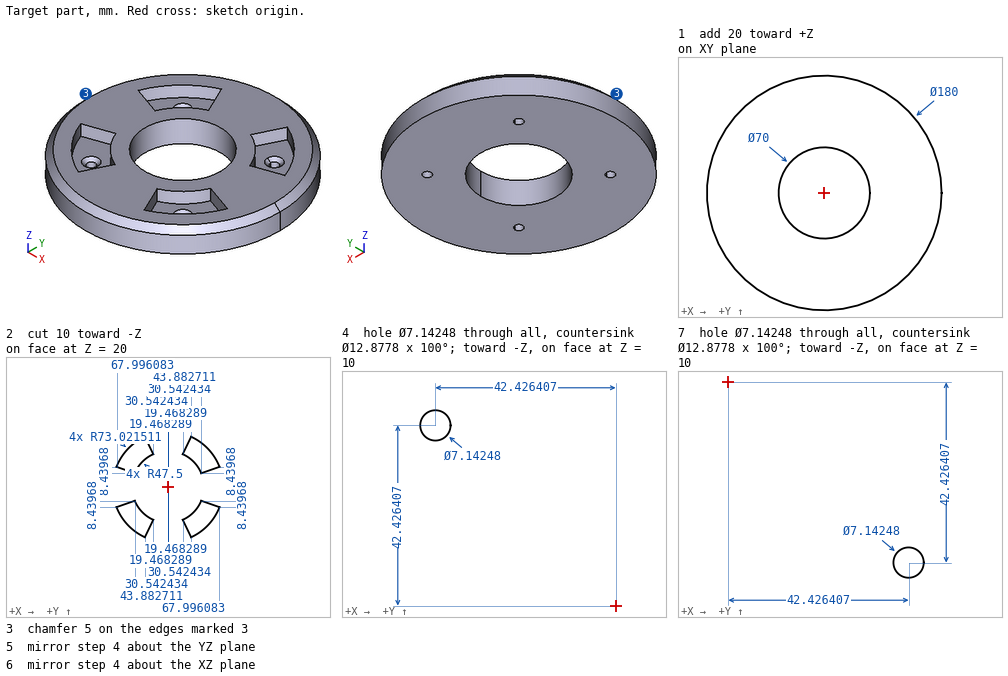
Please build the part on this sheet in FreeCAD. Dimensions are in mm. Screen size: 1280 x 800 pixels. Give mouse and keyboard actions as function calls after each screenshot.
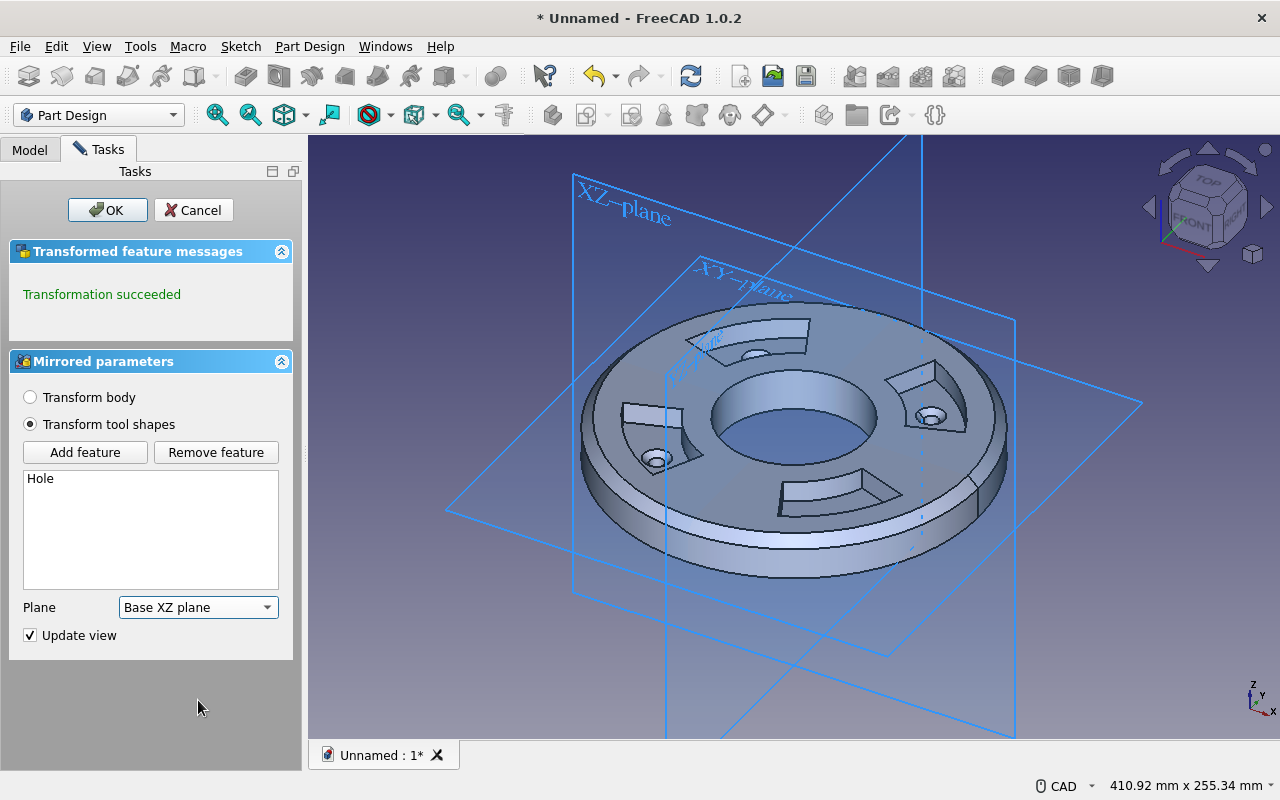
click(108, 210)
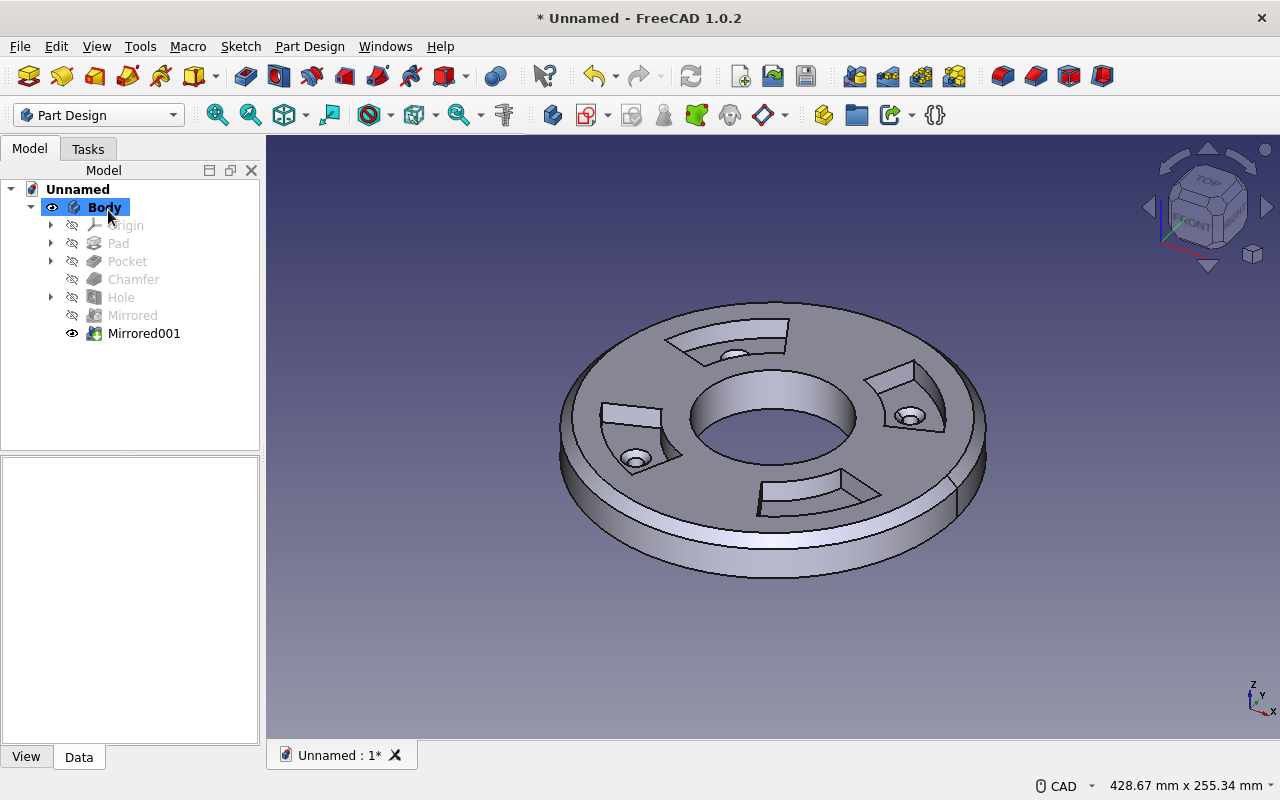
key(0)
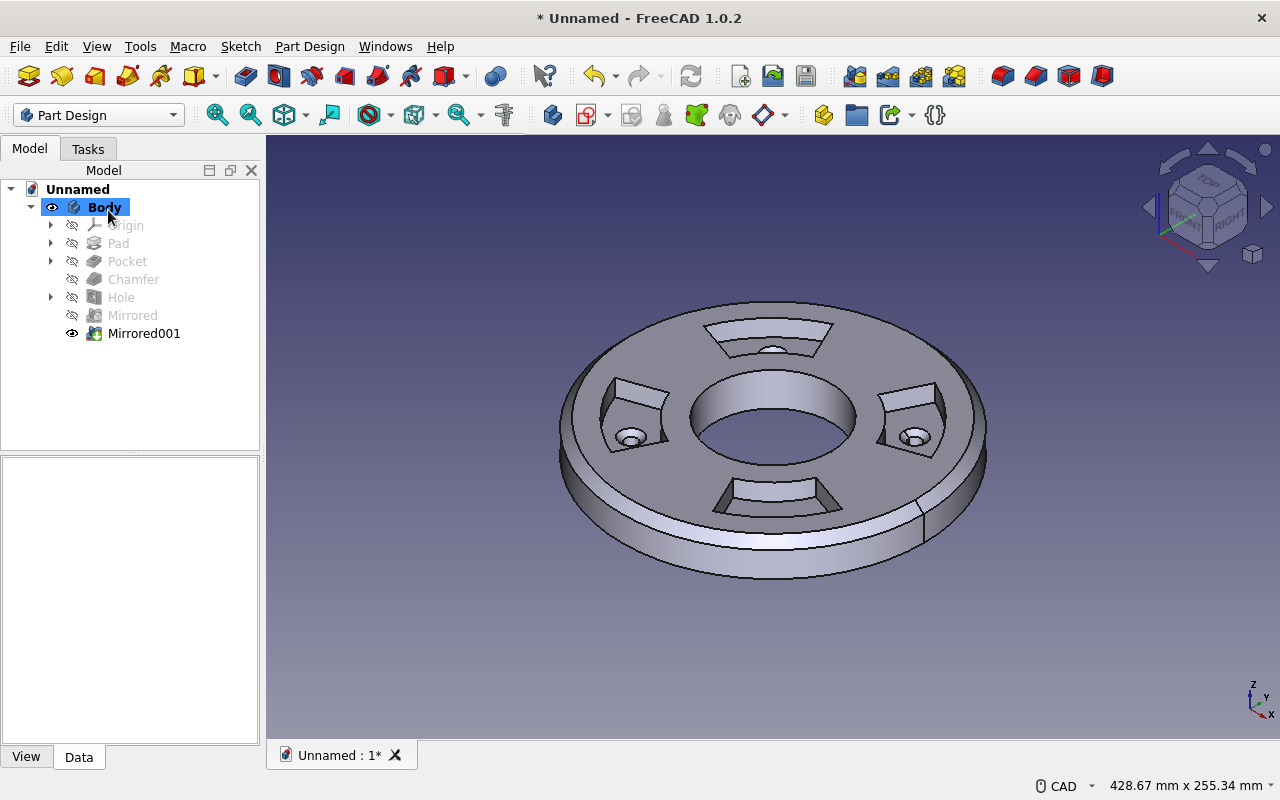
key(2)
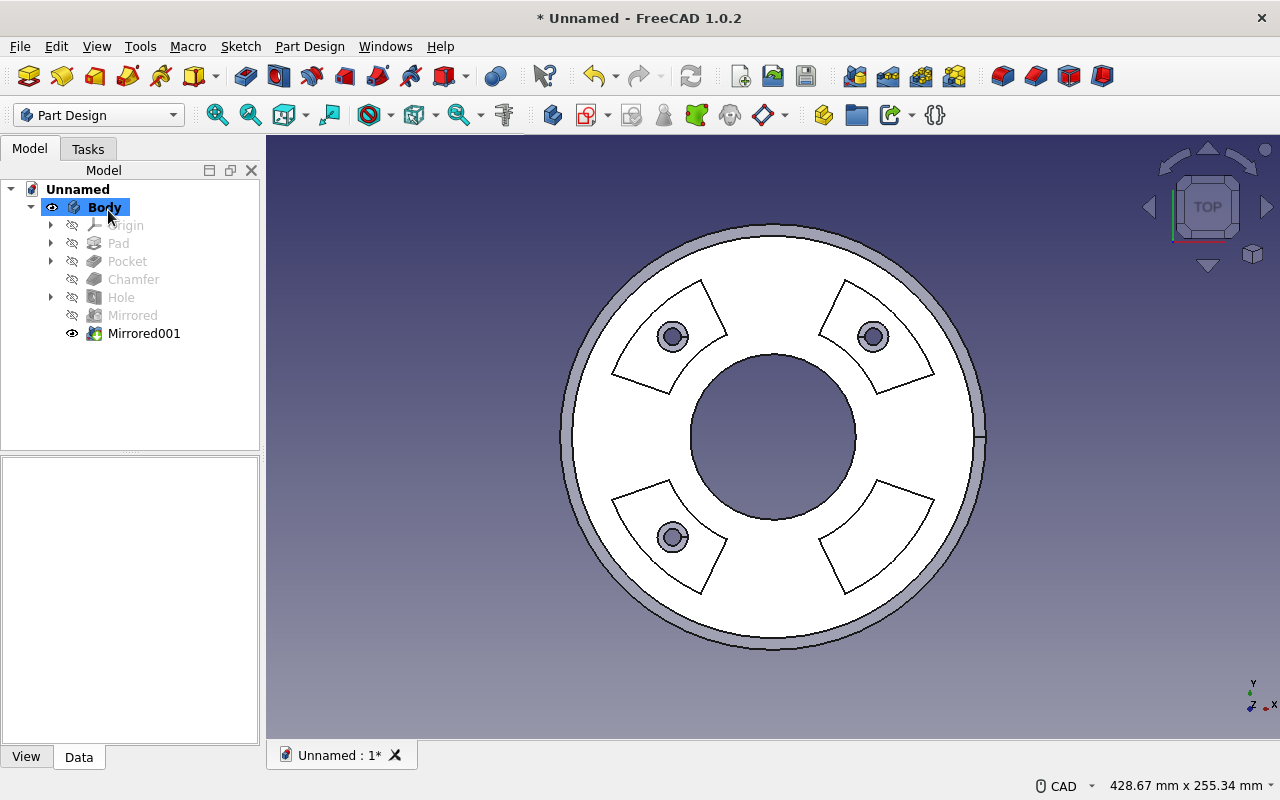
click(876, 536)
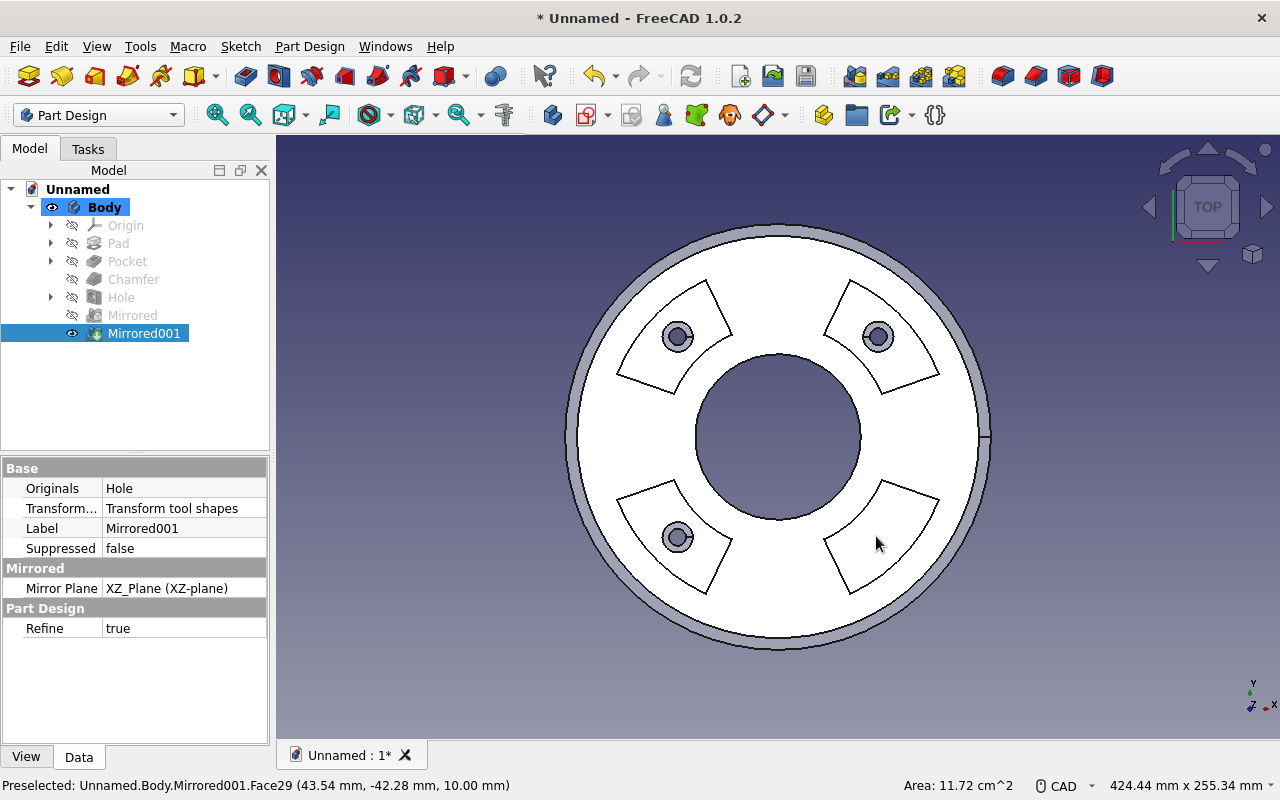
click(586, 116)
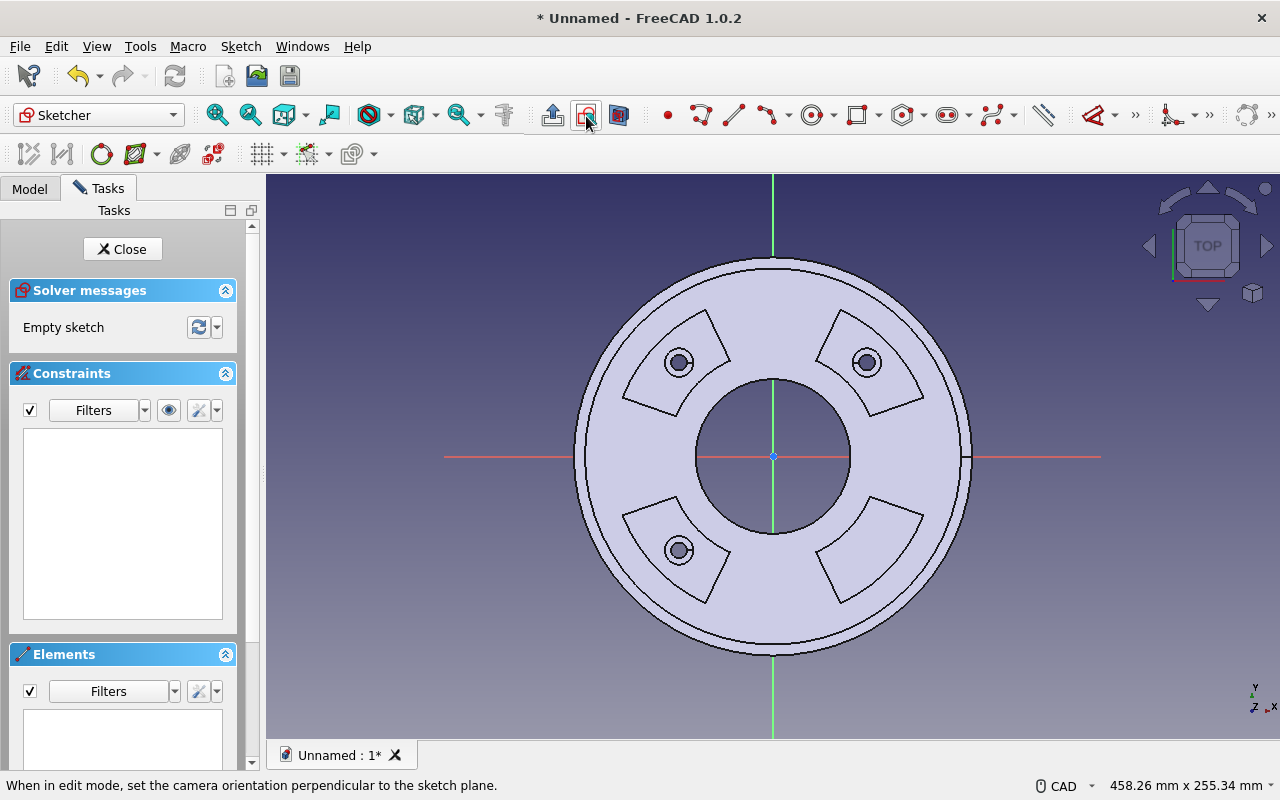
key(q)
key(s)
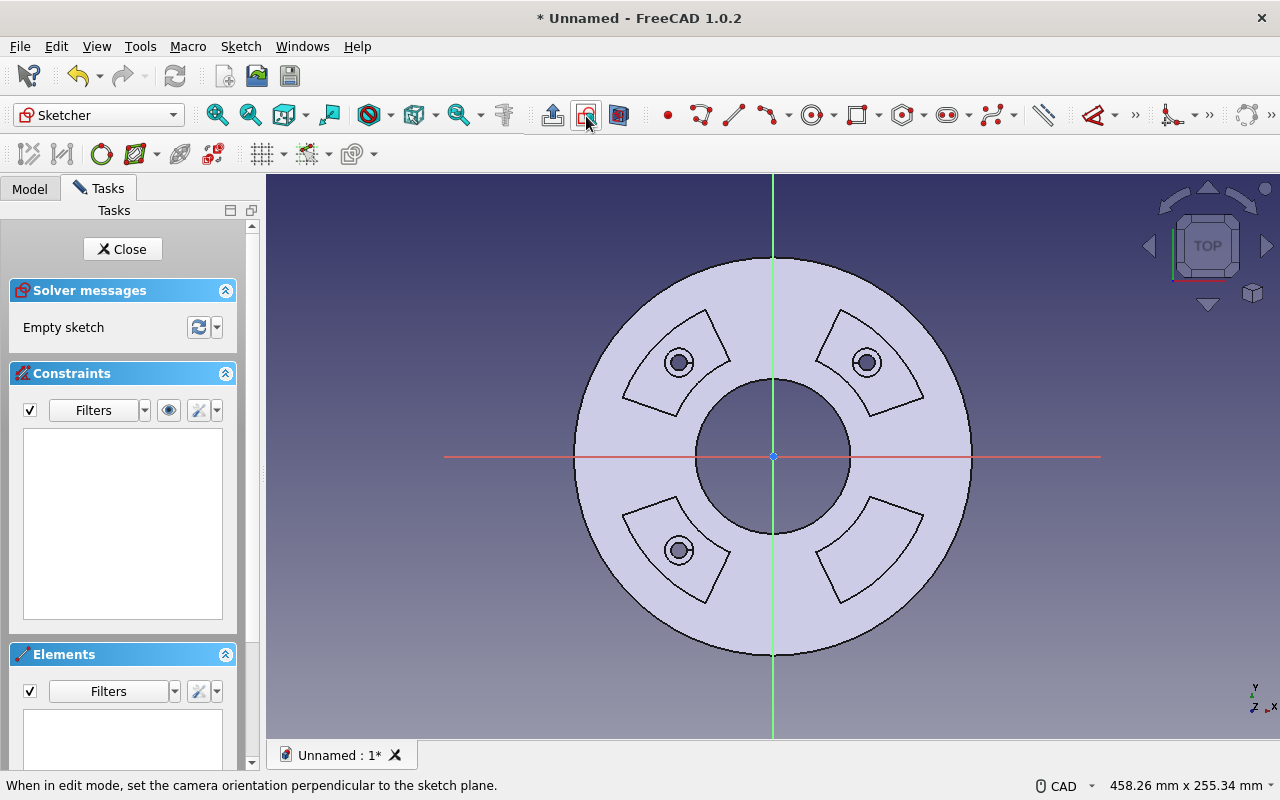
scroll(875, 555, up, 15)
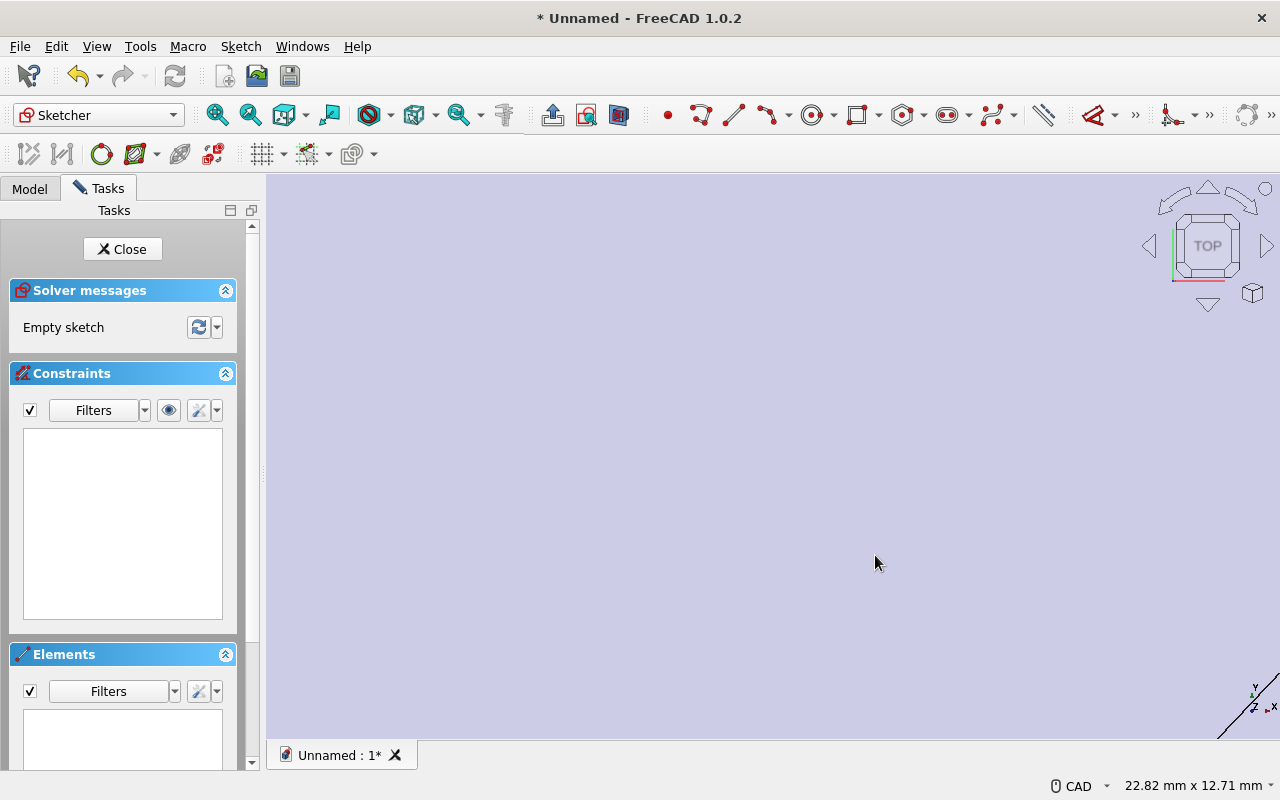
key(g)
key(c)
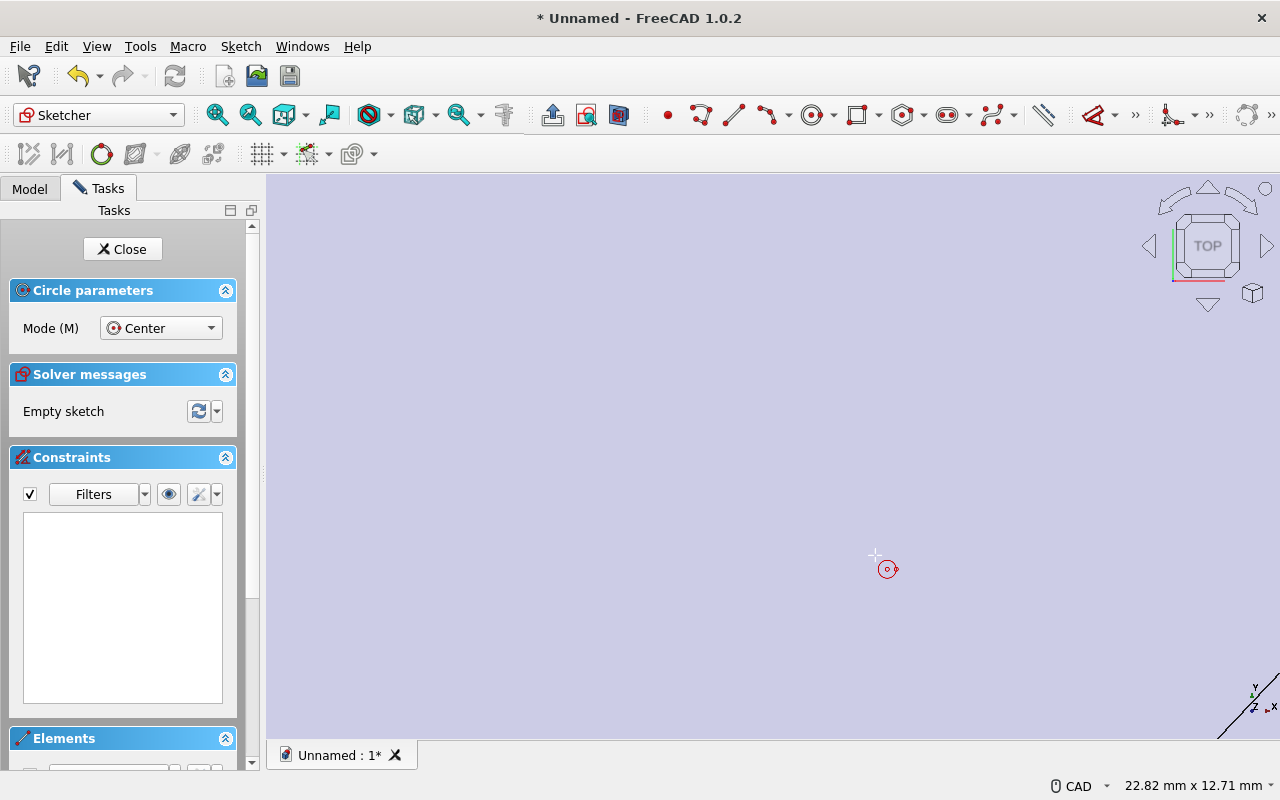
click(700, 449)
move(813, 337)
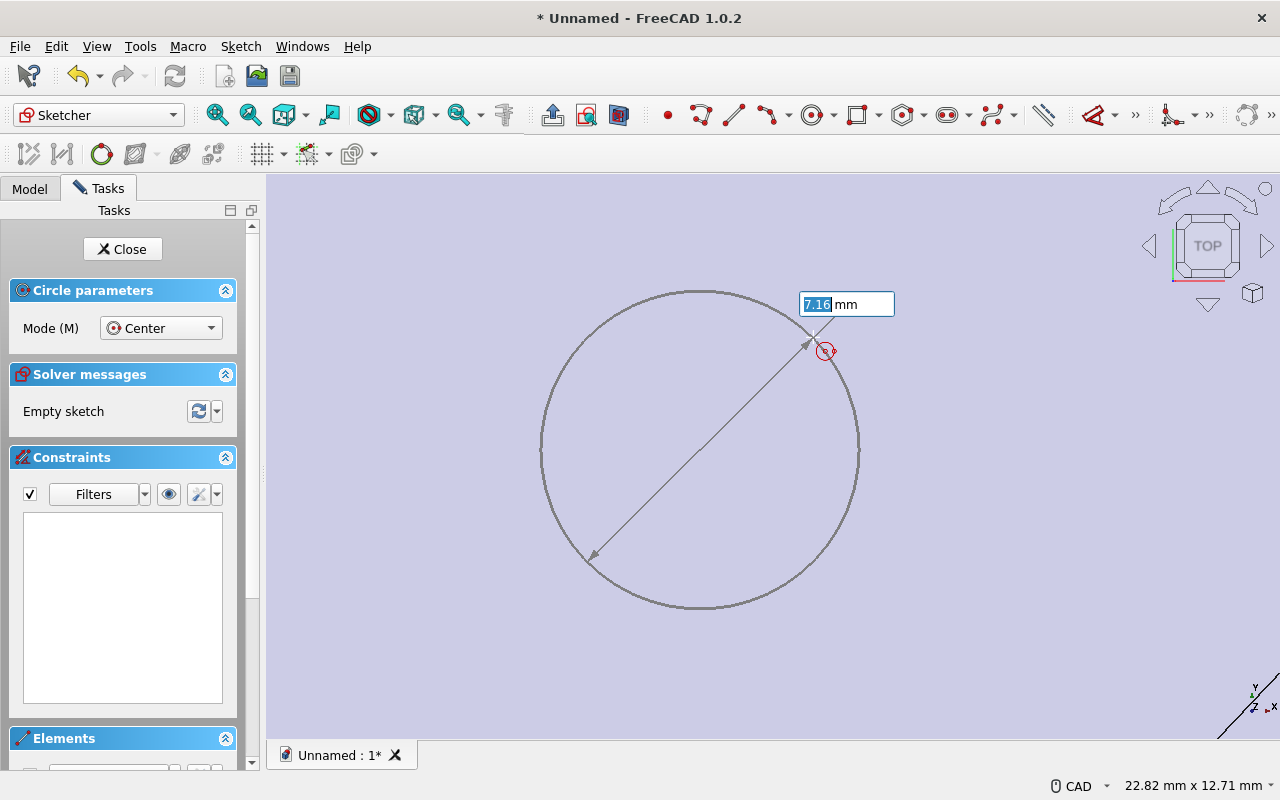
text(7.14248)
key(Return)
key(Escape)